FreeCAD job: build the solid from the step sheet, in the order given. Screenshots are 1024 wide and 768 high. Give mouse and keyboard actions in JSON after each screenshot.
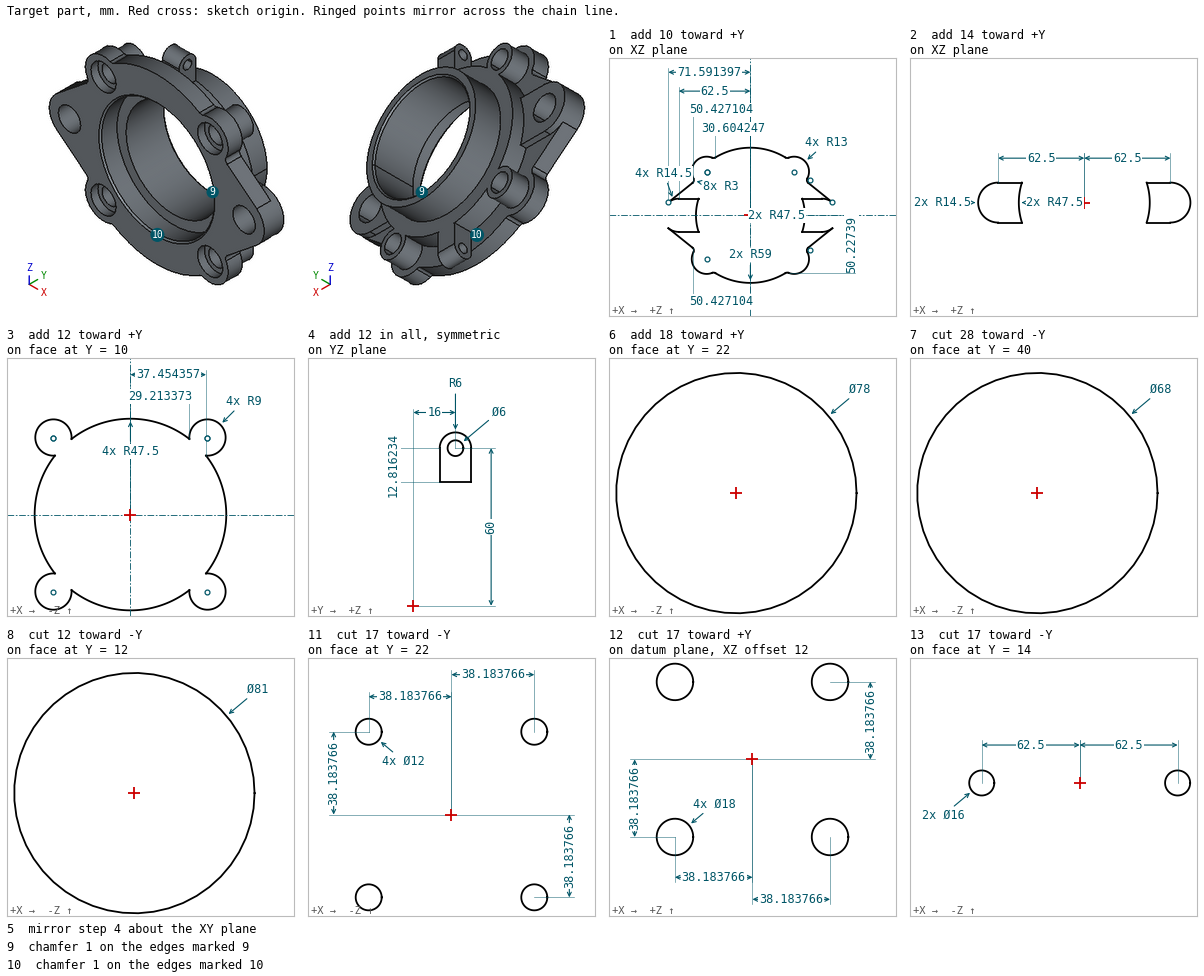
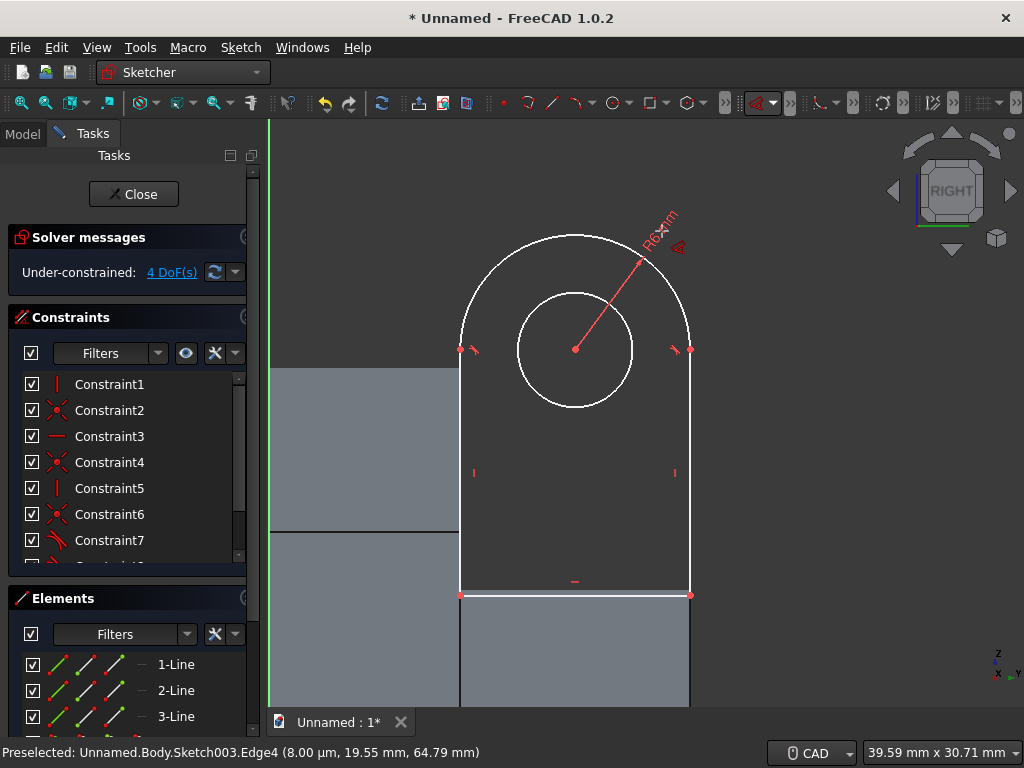
{"action": "left_click", "coordinate": [616, 309]}
{"action": "left_click", "coordinate": [639, 286]}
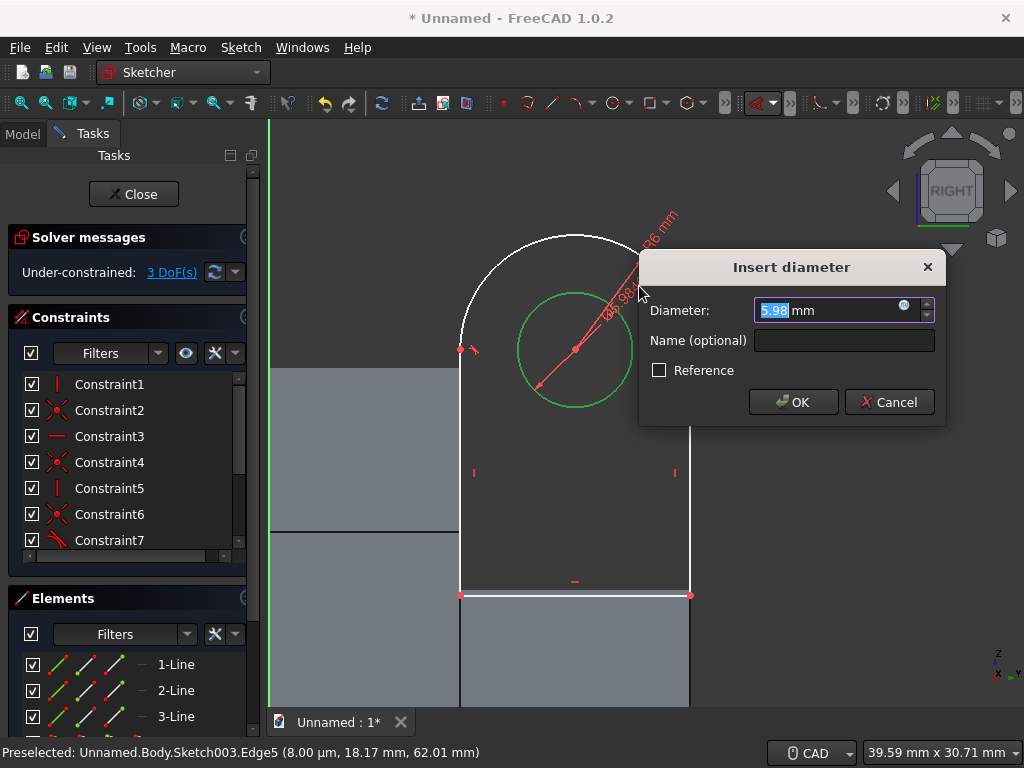
{"action": "type", "text": "6"}
{"action": "key", "text": "Return"}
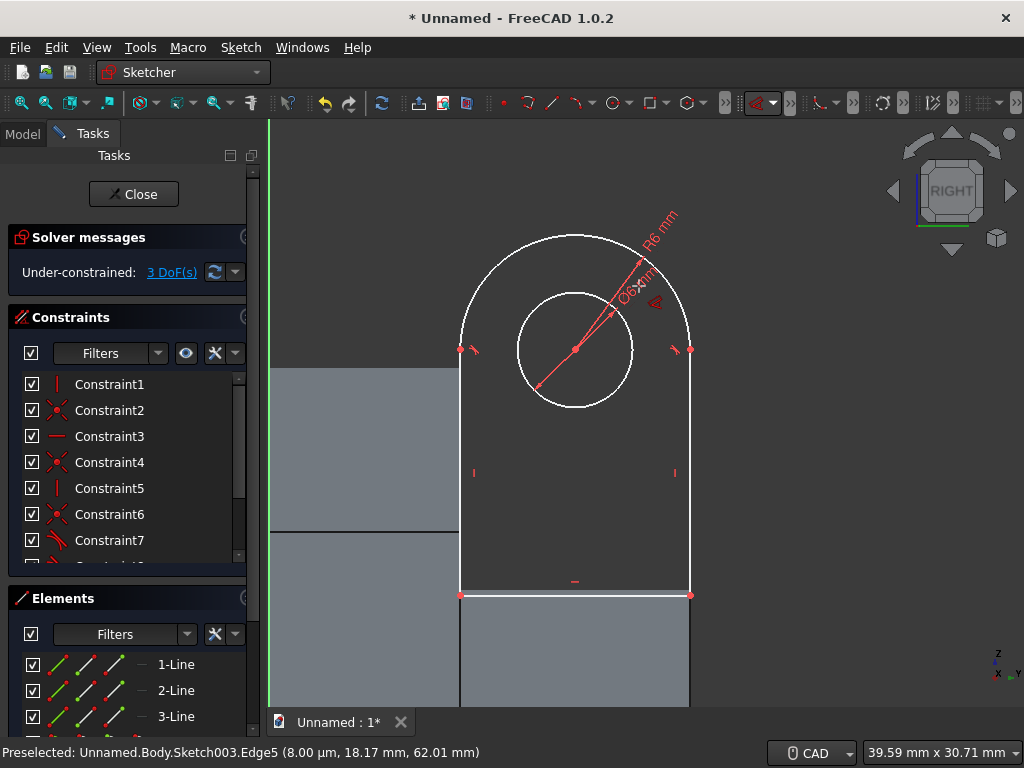
{"action": "left_click", "coordinate": [575, 350]}
{"action": "left_click", "coordinate": [435, 316]}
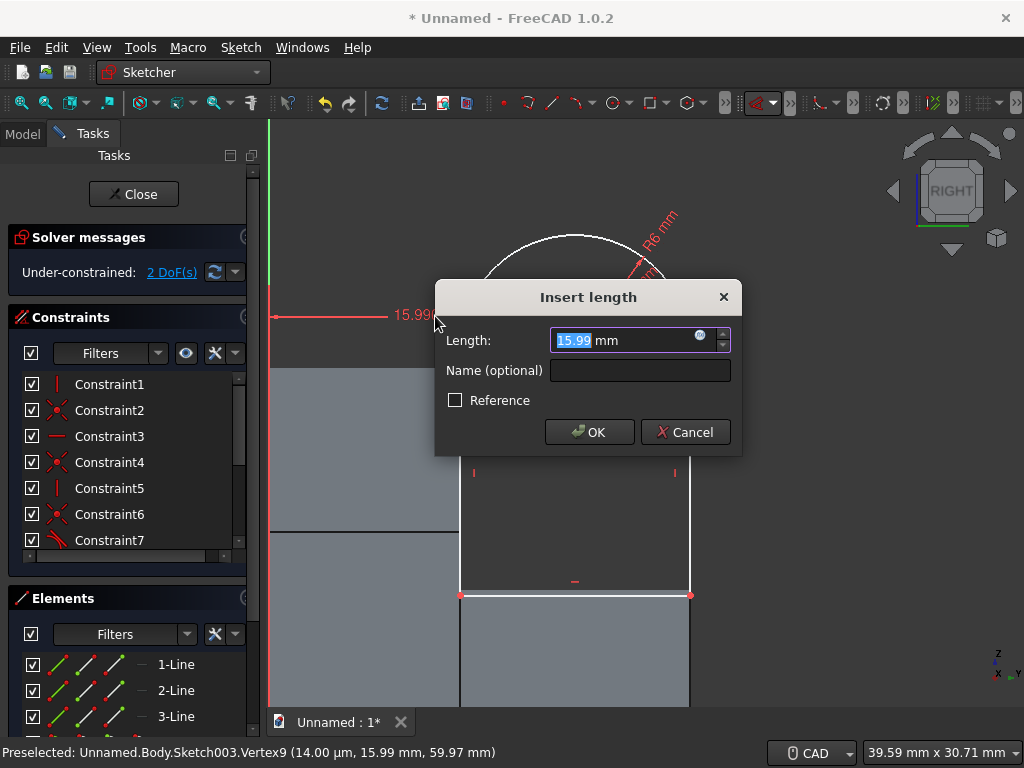
{"action": "type", "text": "16"}
{"action": "key", "text": "Return"}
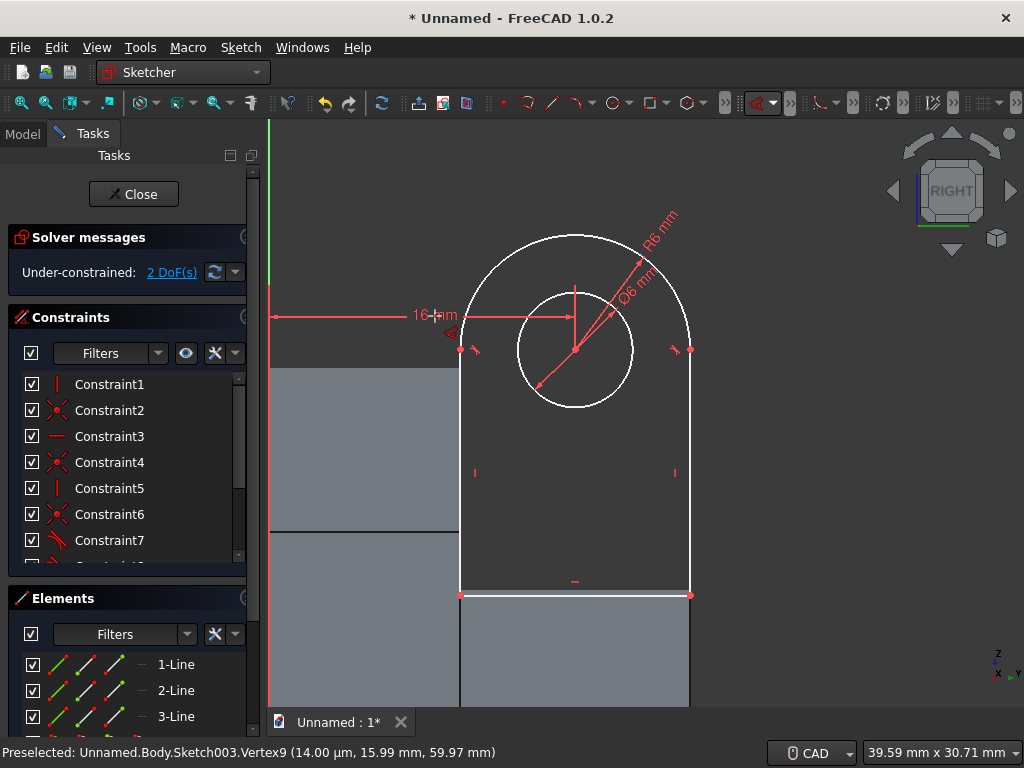
{"action": "left_click", "coordinate": [575, 350]}
{"action": "left_click", "coordinate": [609, 514]}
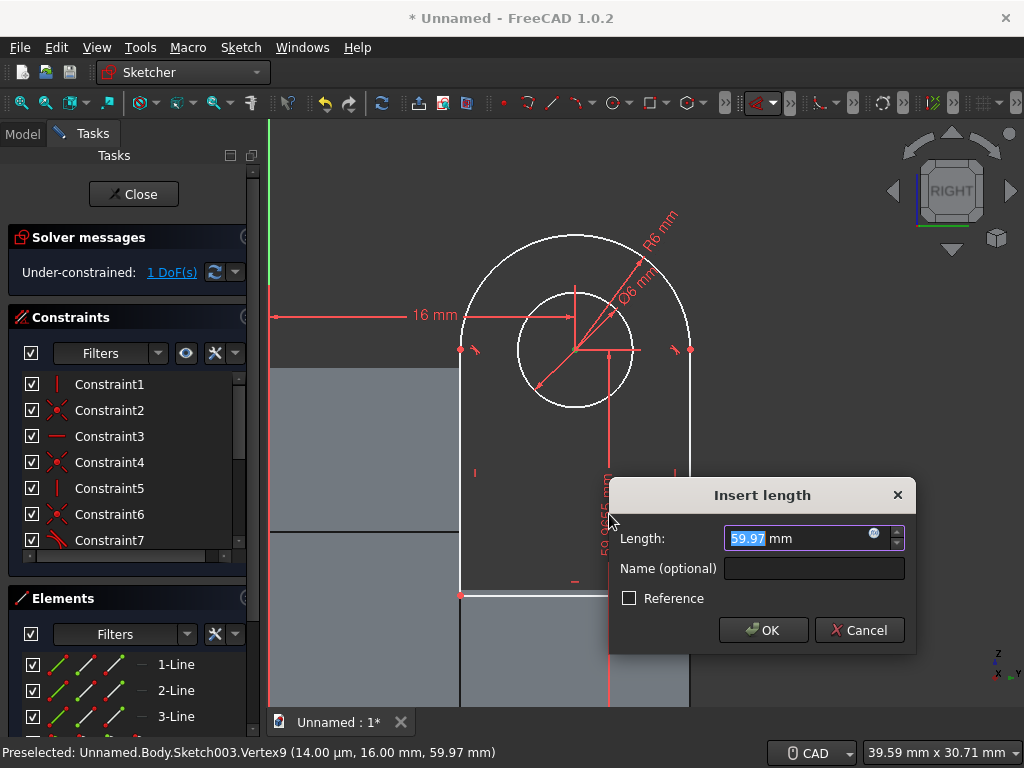
{"action": "type", "text": "60"}
{"action": "key", "text": "Return"}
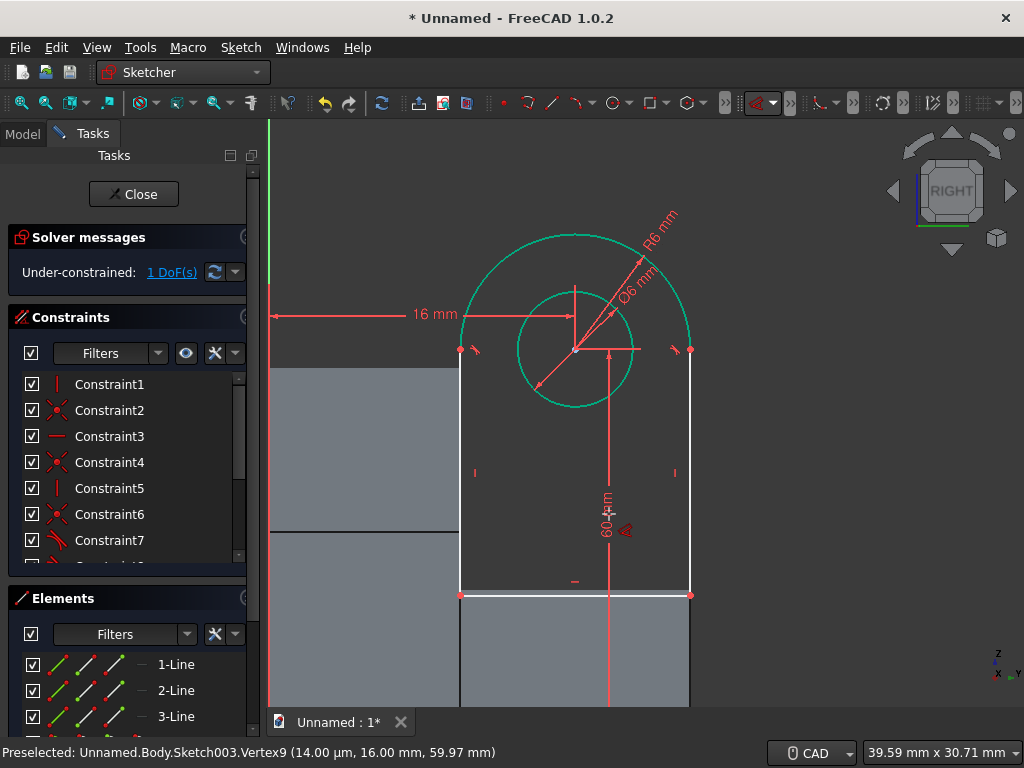
{"action": "left_click", "coordinate": [460, 423]}
{"action": "left_click", "coordinate": [426, 473]}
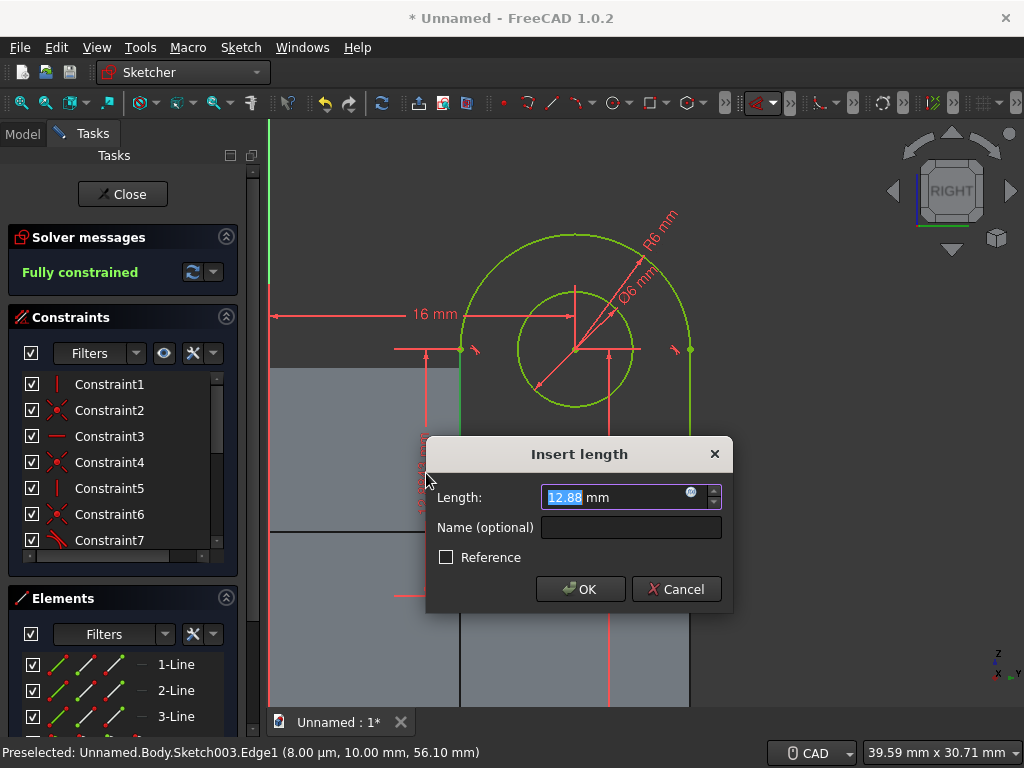
{"action": "type", "text": "12.816234"}
{"action": "key", "text": "Return"}
{"action": "key", "text": "Escape"}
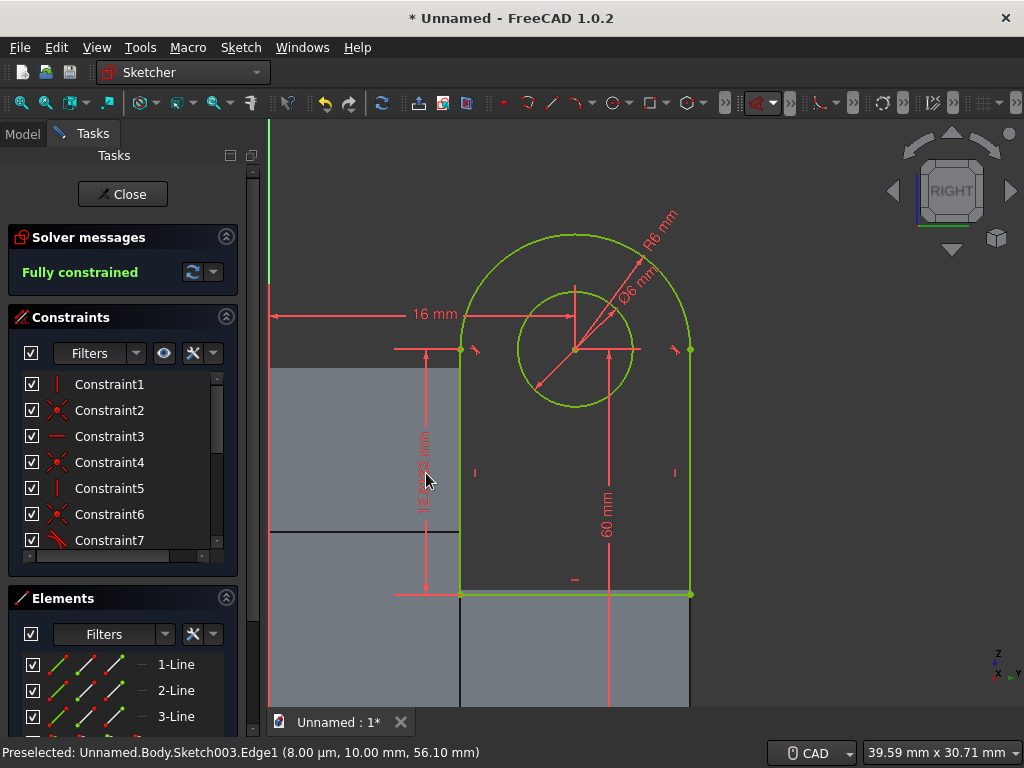
{"action": "left_click", "coordinate": [123, 194]}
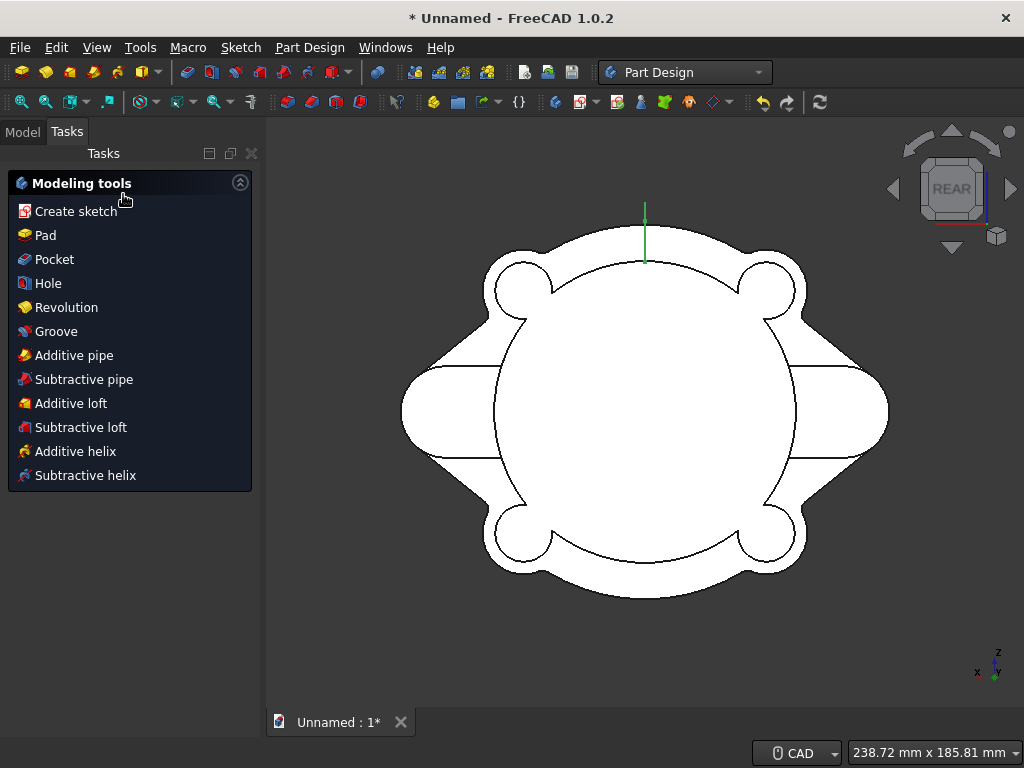
{"action": "left_click", "coordinate": [22, 72]}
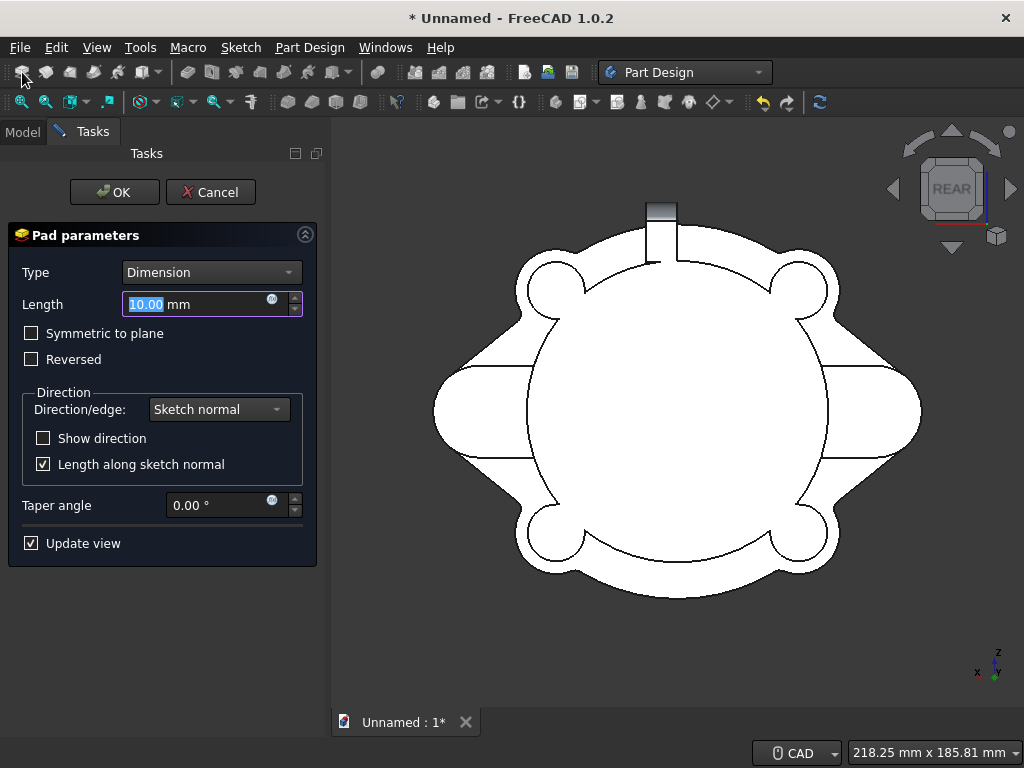
{"action": "type", "text": "12"}
{"action": "key", "text": "Tab"}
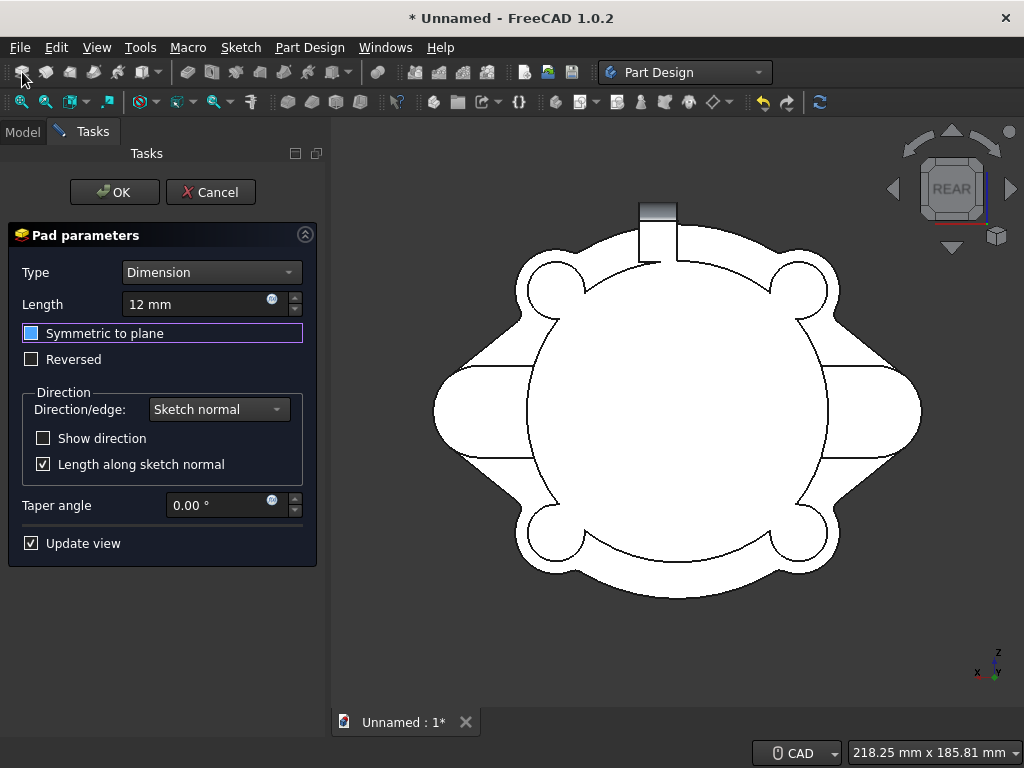
{"action": "left_click", "coordinate": [30, 333]}